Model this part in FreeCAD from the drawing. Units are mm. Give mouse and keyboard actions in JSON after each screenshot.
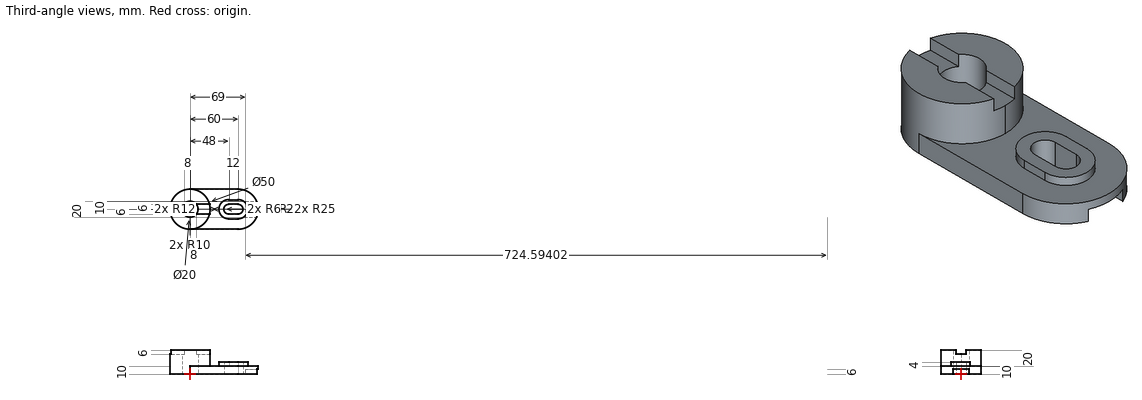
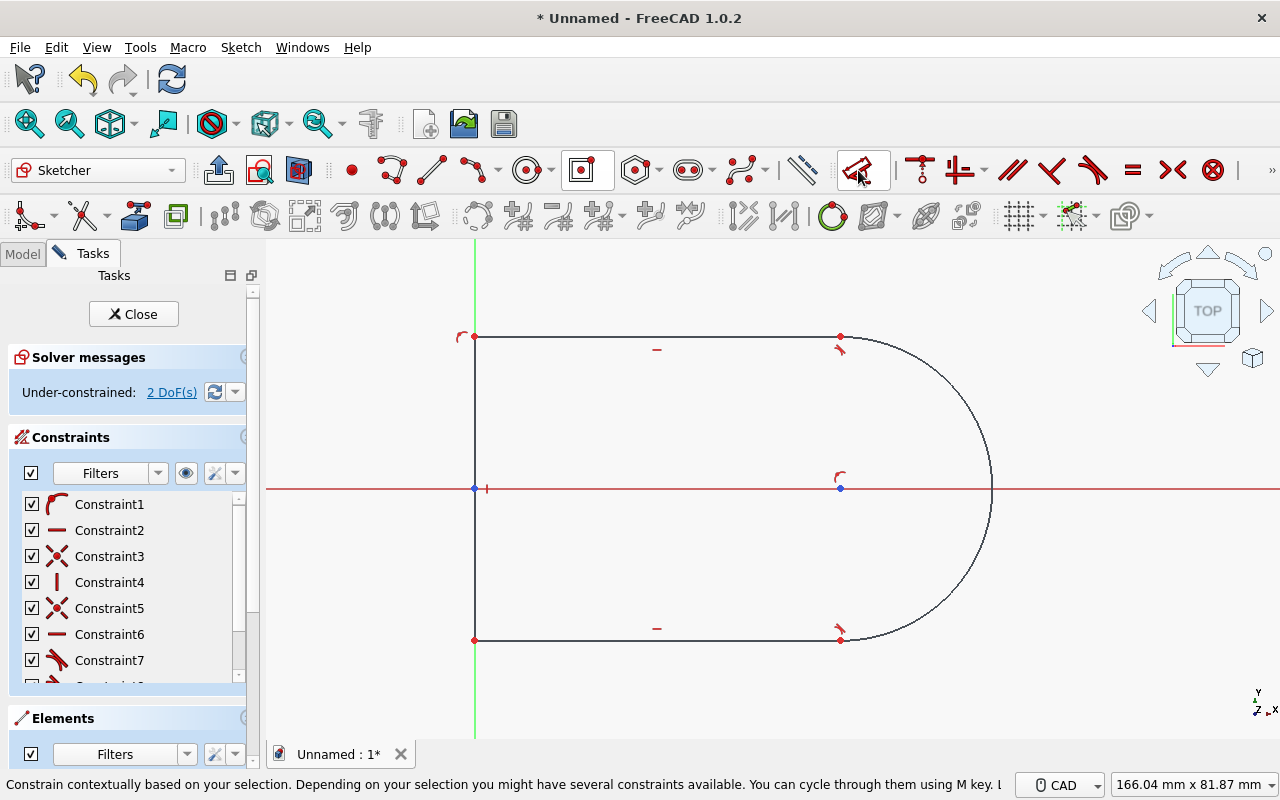
{"action": "left_click", "coordinate": [963, 578]}
{"action": "left_click", "coordinate": [989, 597]}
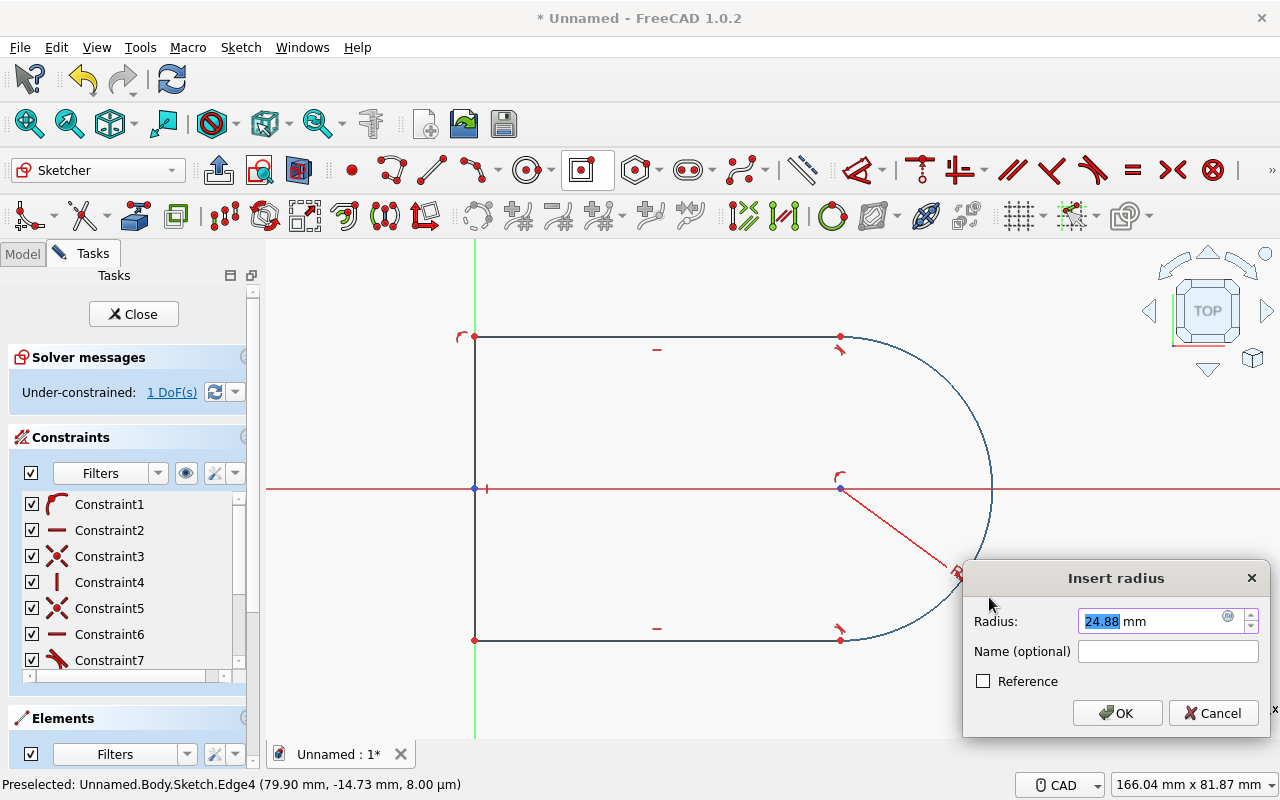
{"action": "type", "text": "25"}
{"action": "key", "text": "Return"}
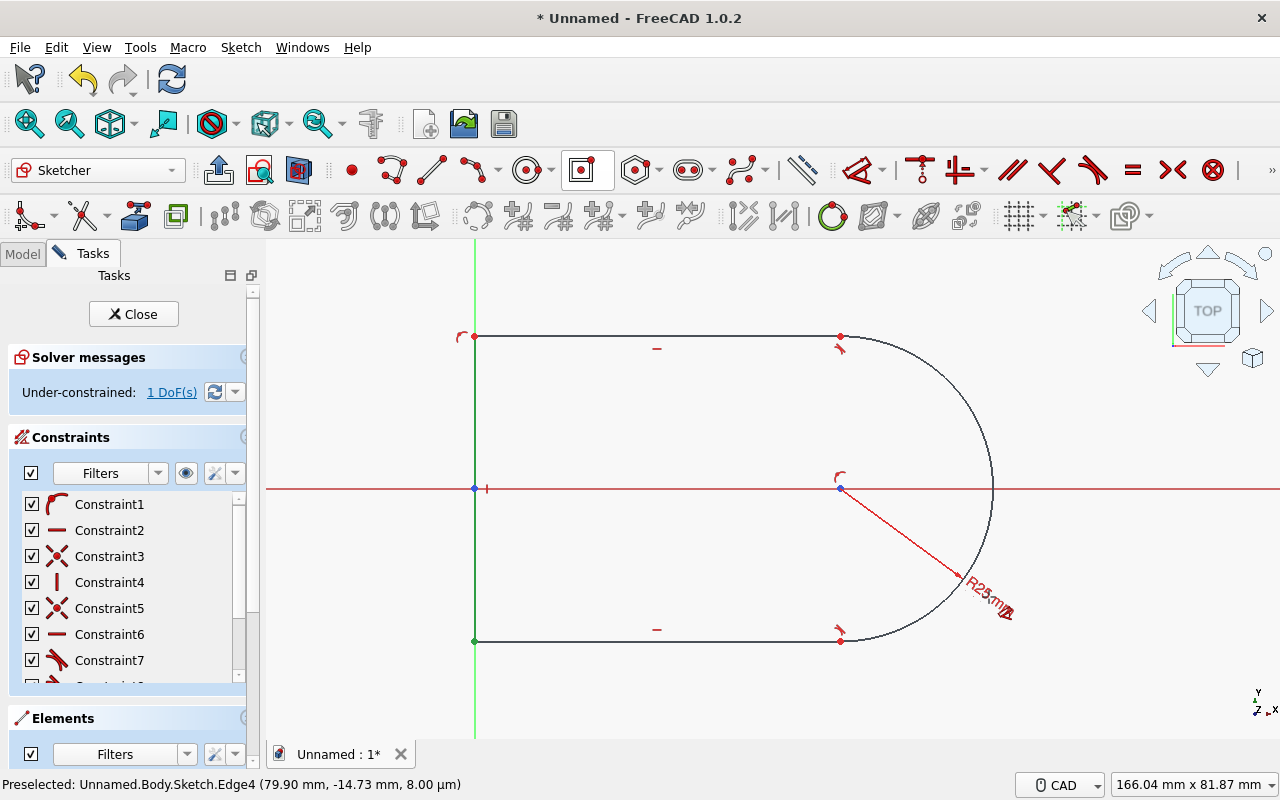
{"action": "left_click", "coordinate": [731, 336]}
{"action": "left_click", "coordinate": [658, 302]}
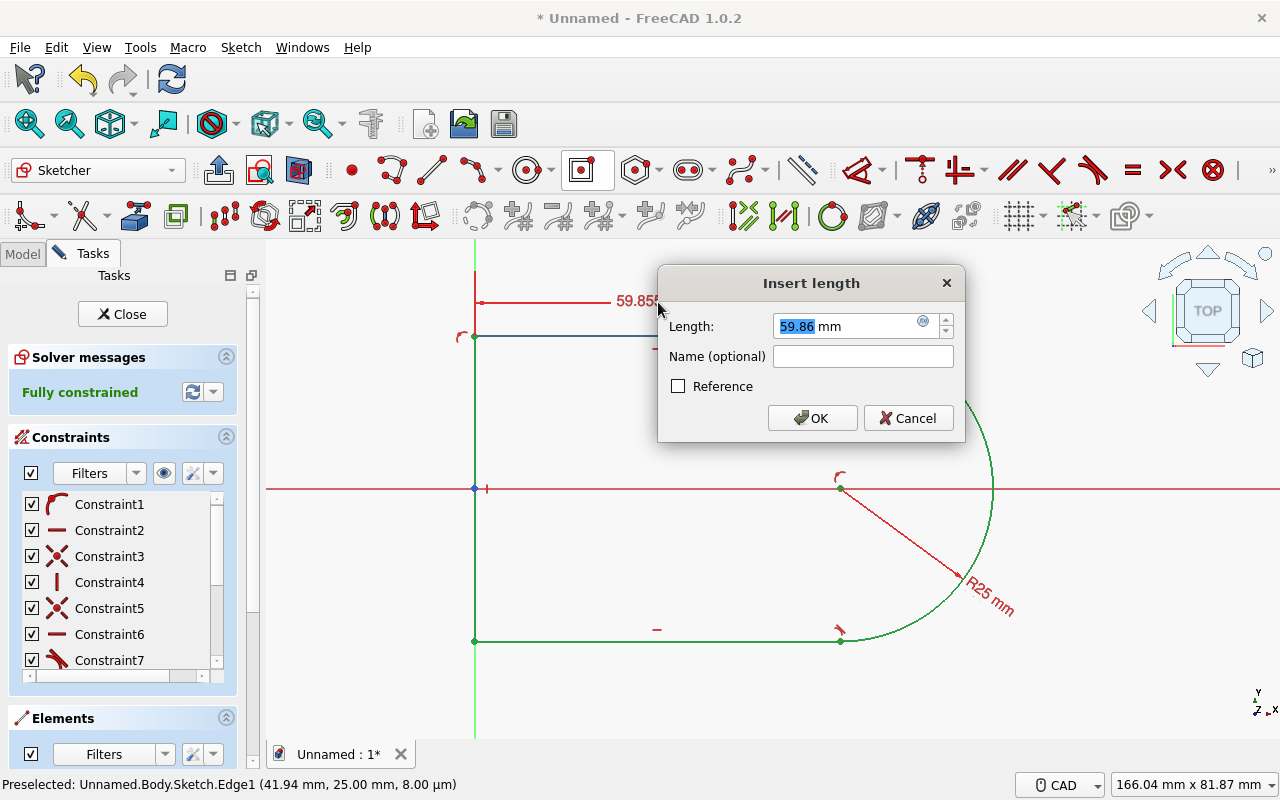
{"action": "type", "text": "60"}
{"action": "key", "text": "Return"}
{"action": "key", "text": "Escape"}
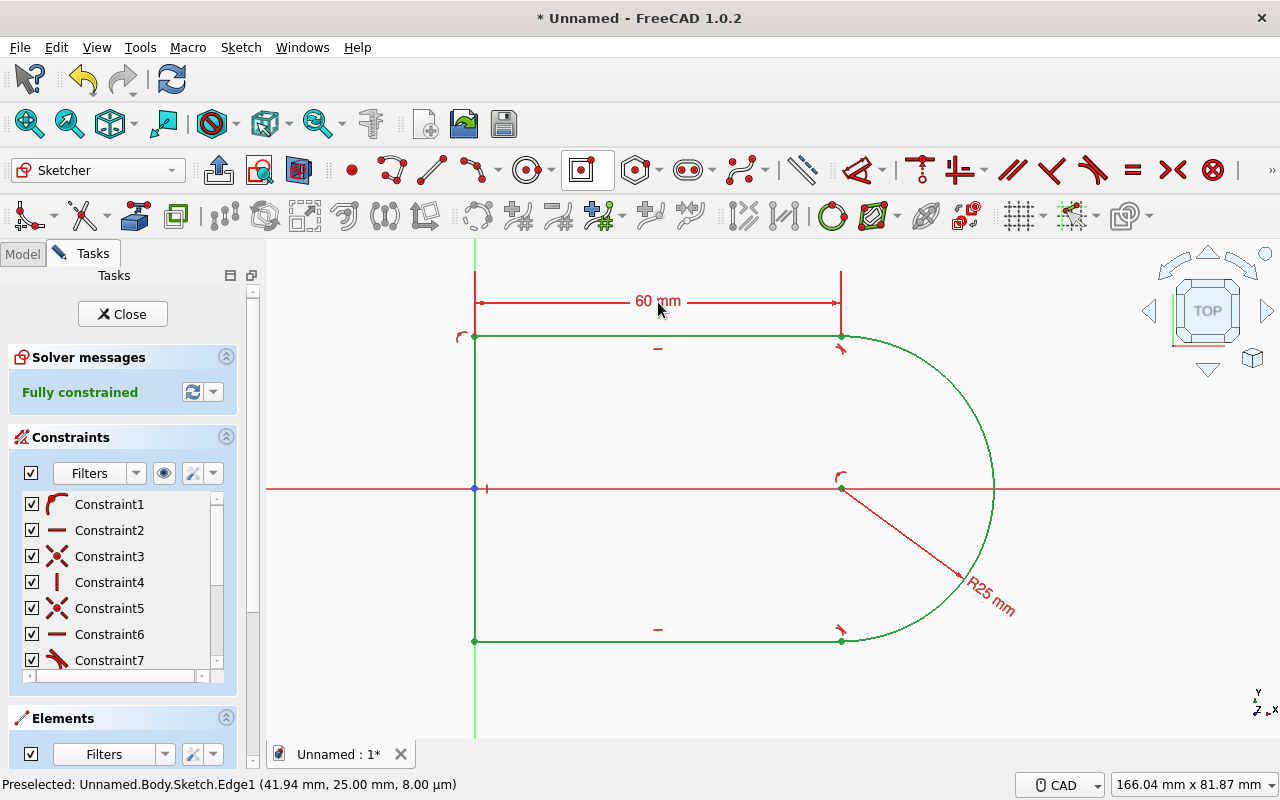
{"action": "left_click", "coordinate": [123, 314]}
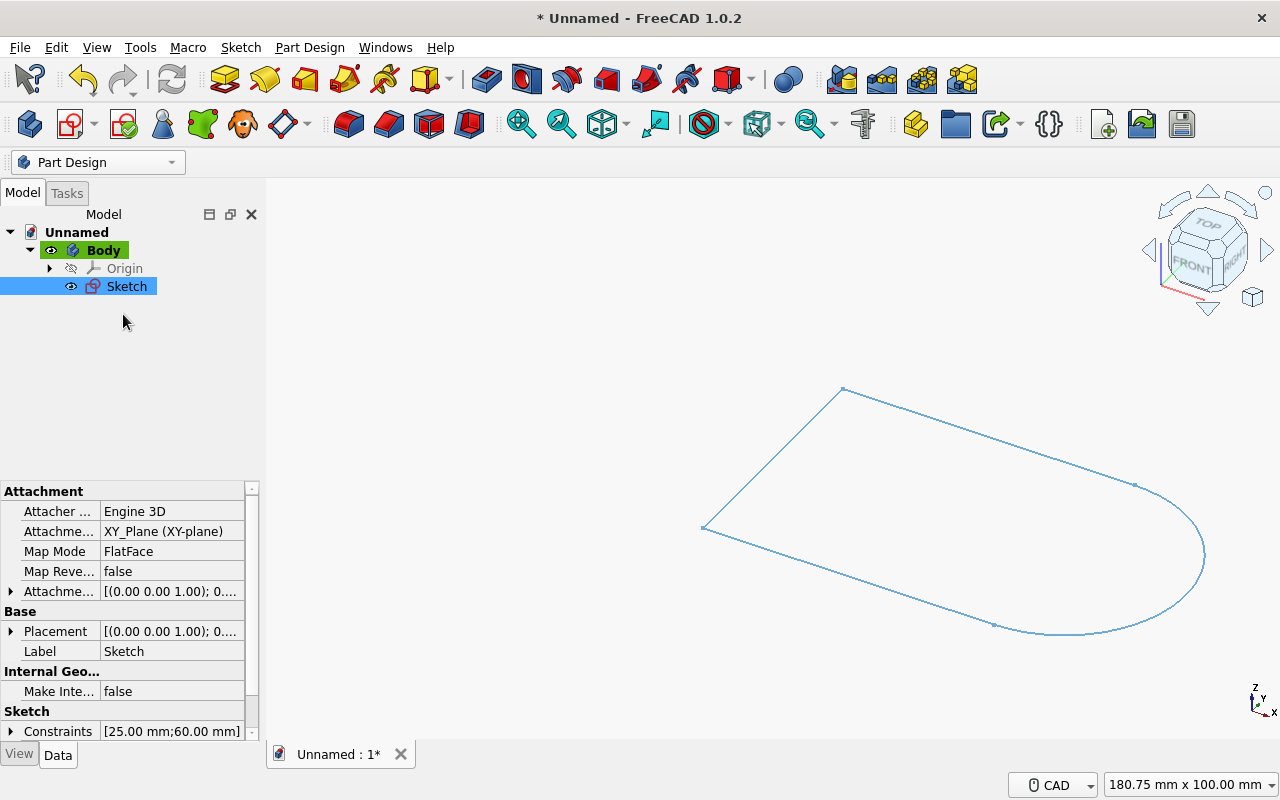
{"action": "left_click", "coordinate": [226, 80]}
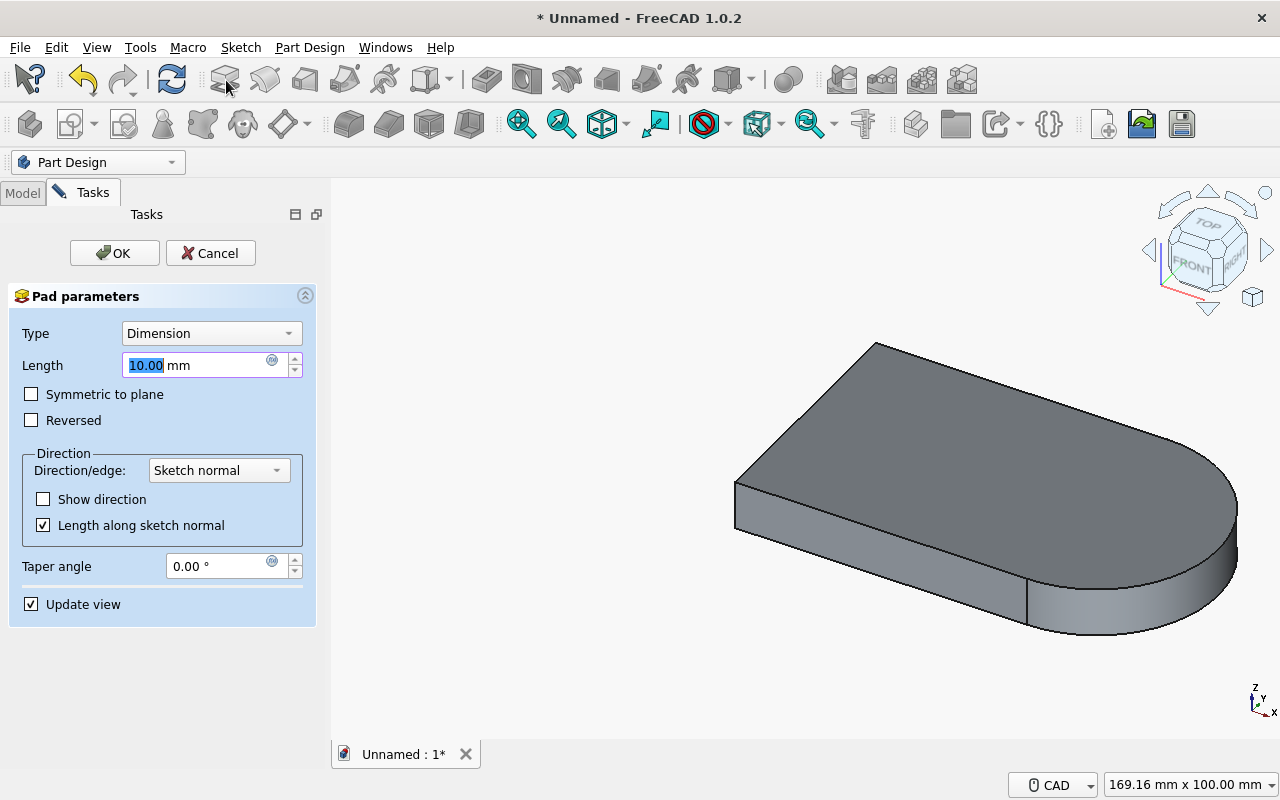
{"action": "type", "text": "10"}
{"action": "key", "text": "Tab"}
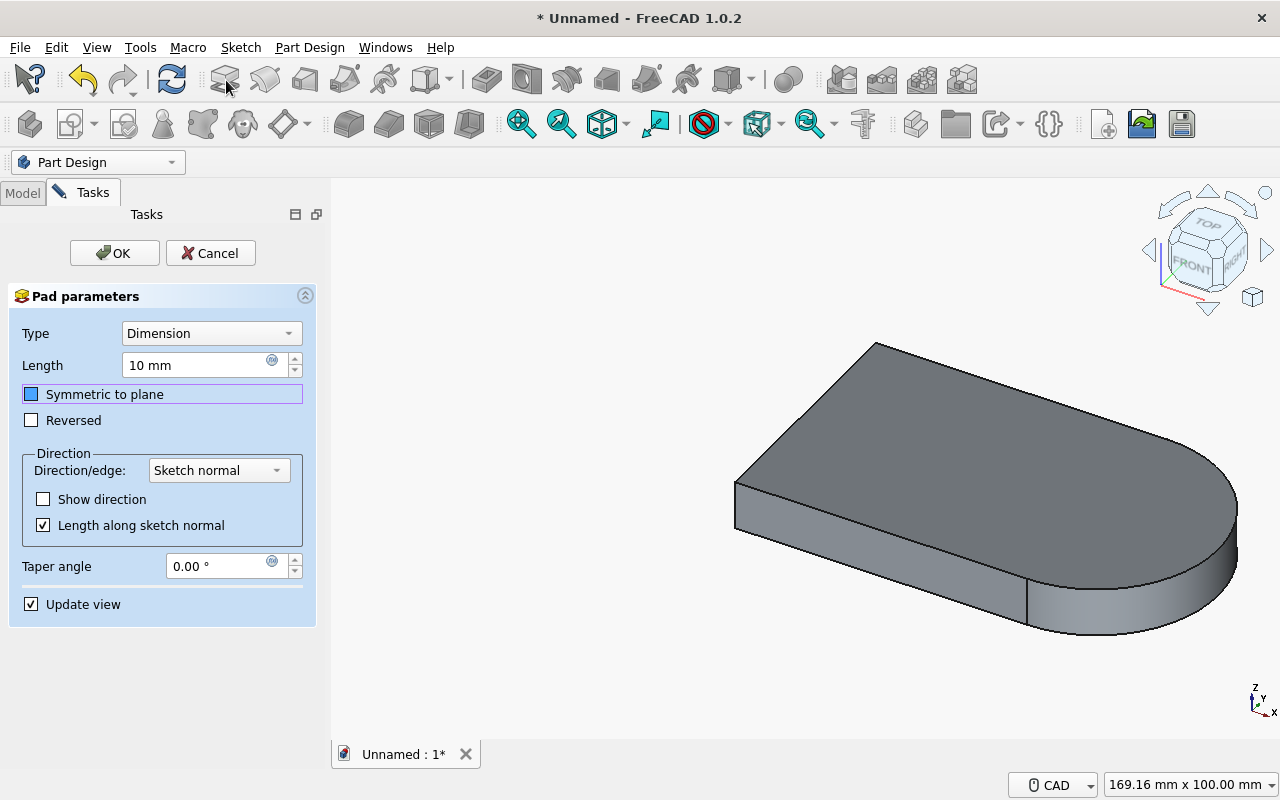
{"action": "left_click", "coordinate": [115, 253]}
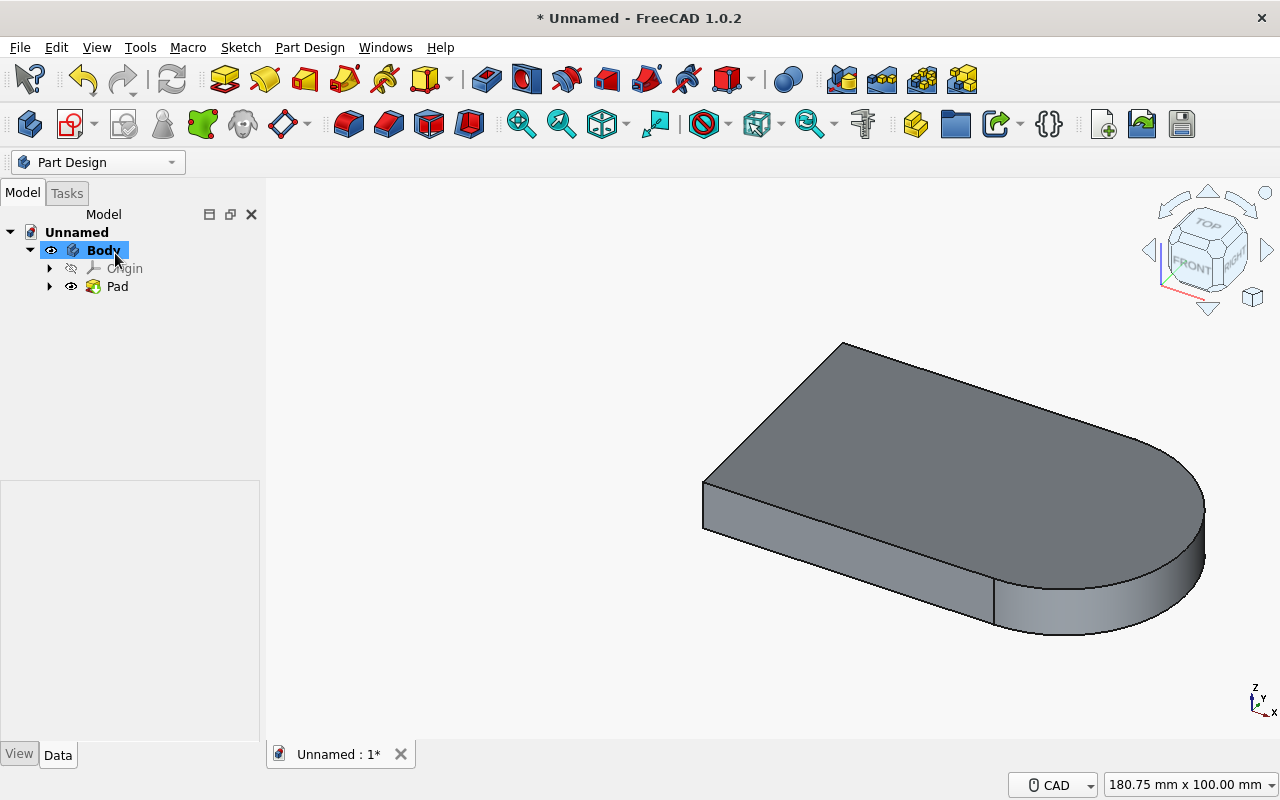
{"action": "left_click", "coordinate": [1038, 499]}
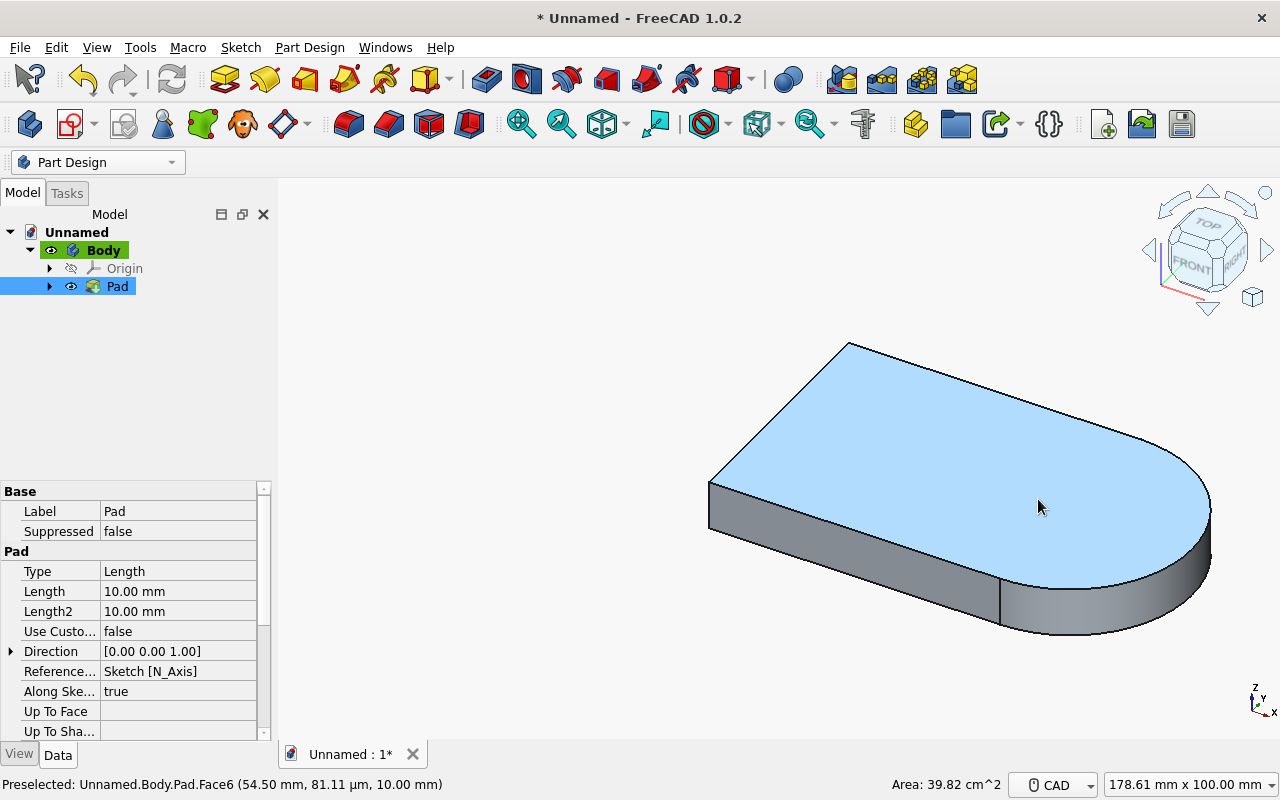
{"action": "left_click", "coordinate": [70, 124]}